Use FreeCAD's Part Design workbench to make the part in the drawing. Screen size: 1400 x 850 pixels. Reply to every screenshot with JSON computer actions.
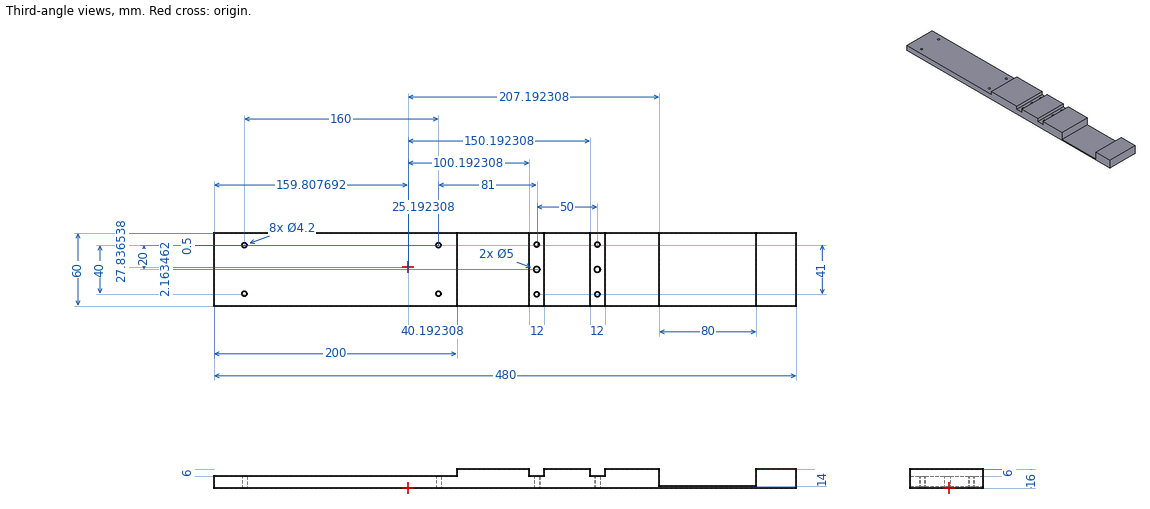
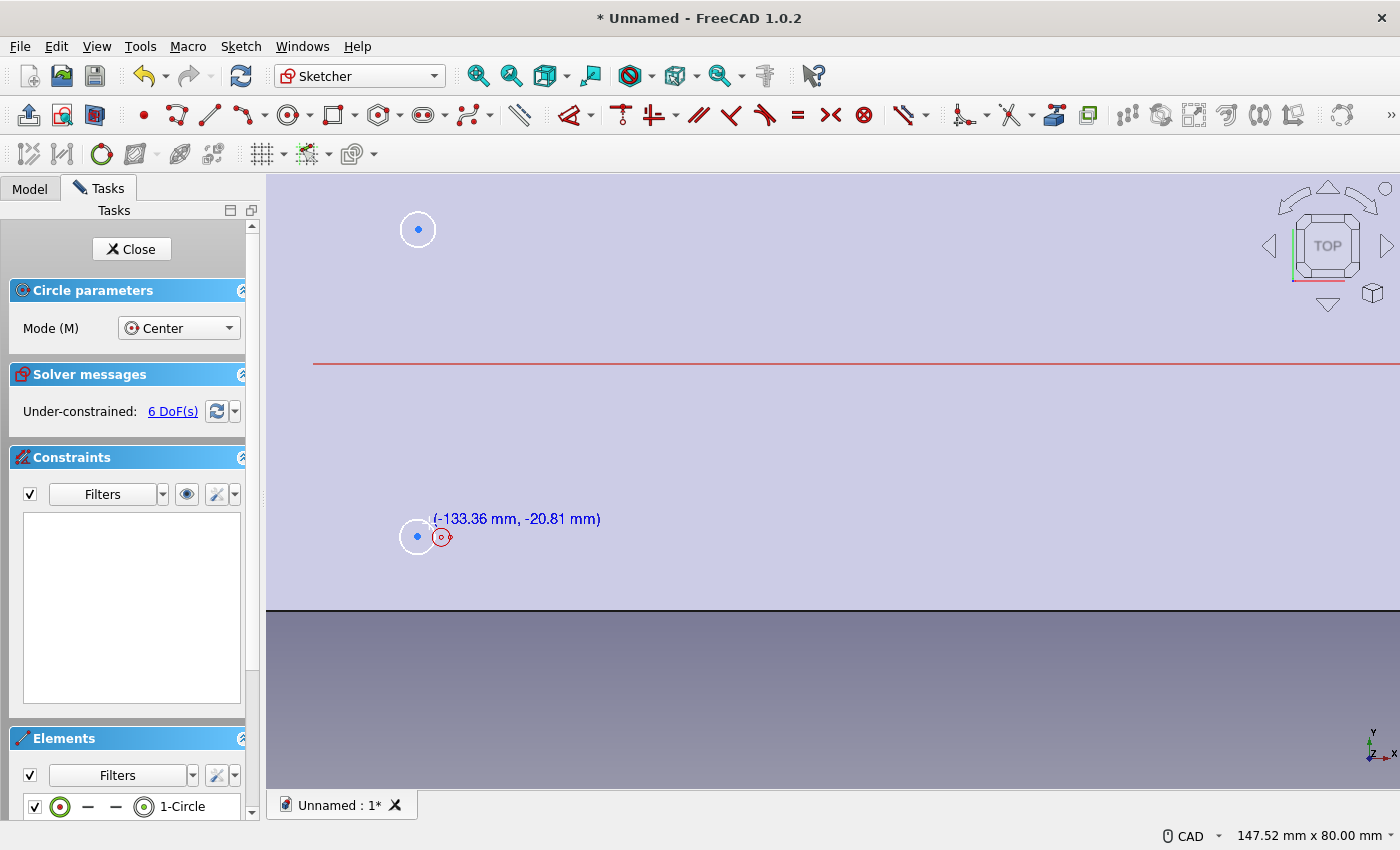
{"action": "scroll", "coordinate": [431, 525], "scroll_direction": "down", "scroll_amount": 6}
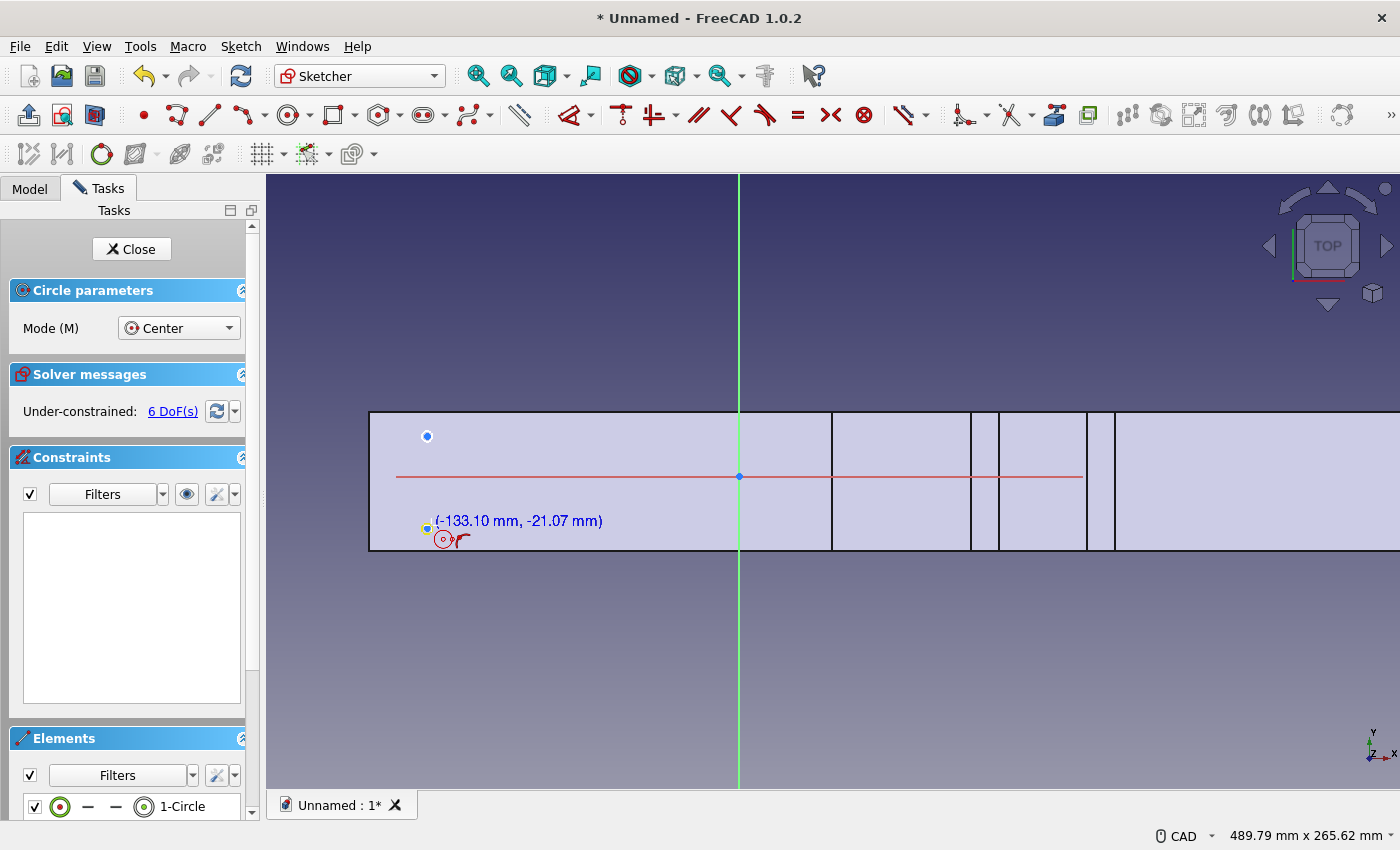
{"action": "scroll", "coordinate": [798, 436], "scroll_direction": "up", "scroll_amount": 8}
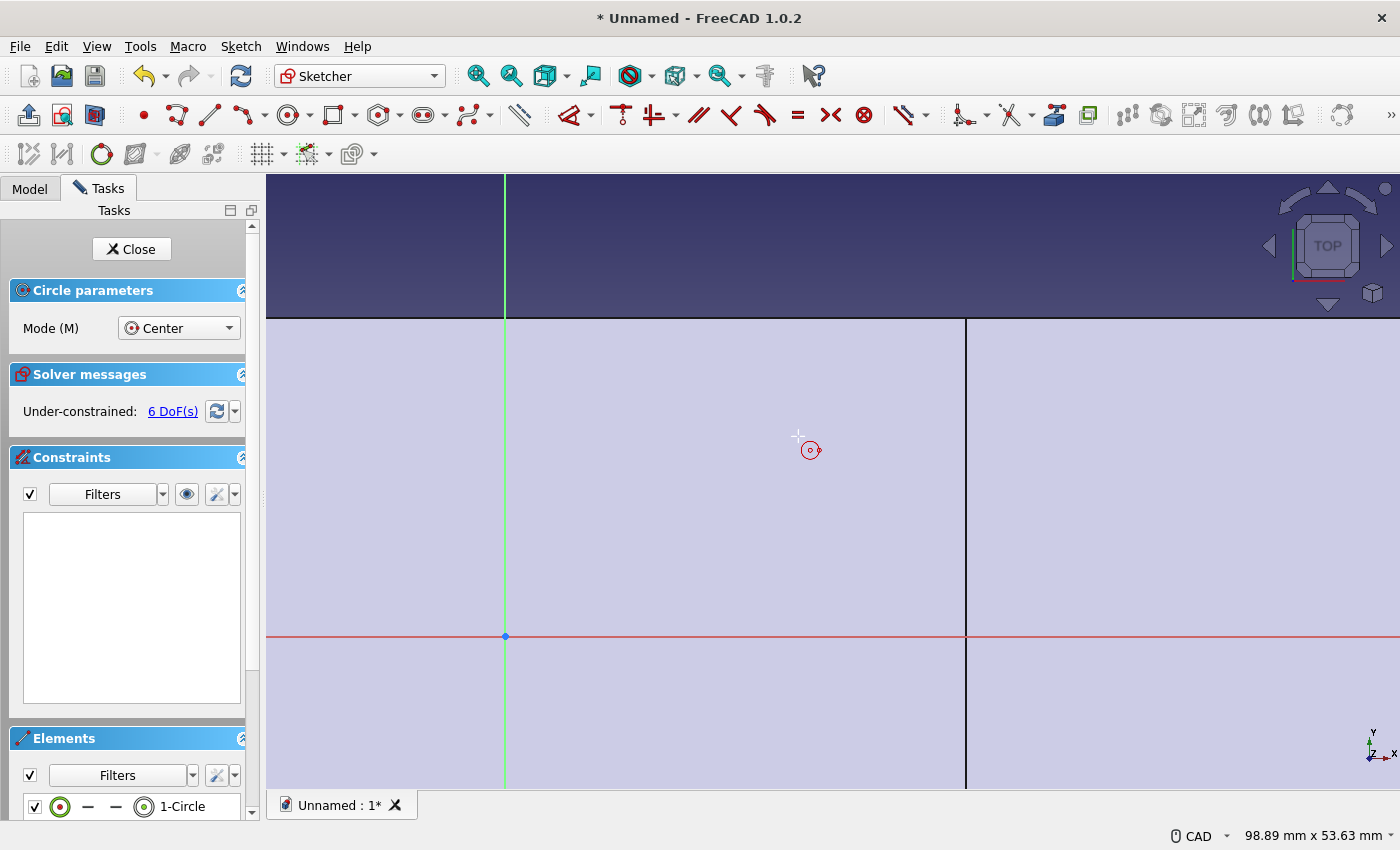
{"action": "scroll", "coordinate": [798, 436], "scroll_direction": "down", "scroll_amount": 8}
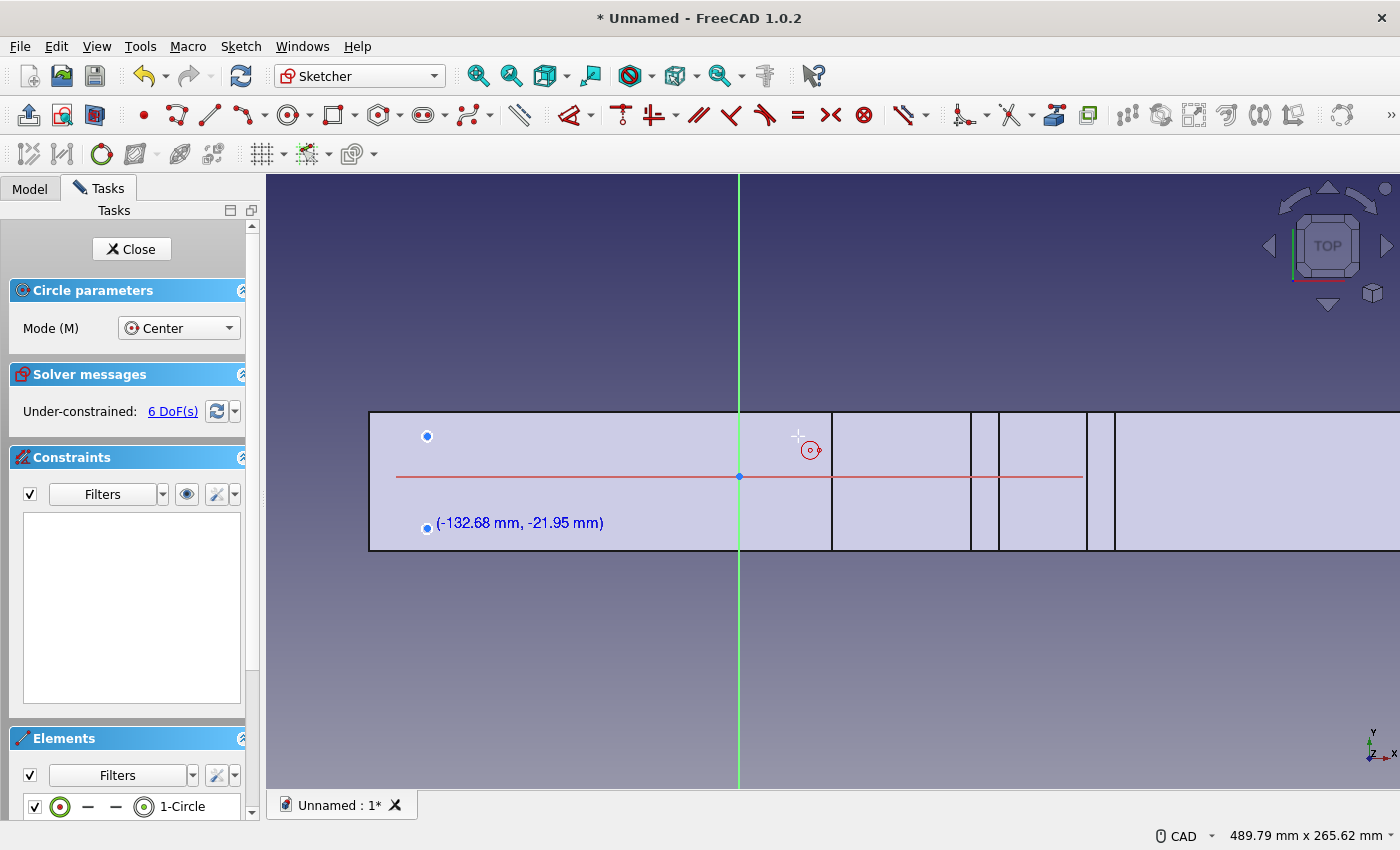
{"action": "left_click", "coordinate": [798, 436]}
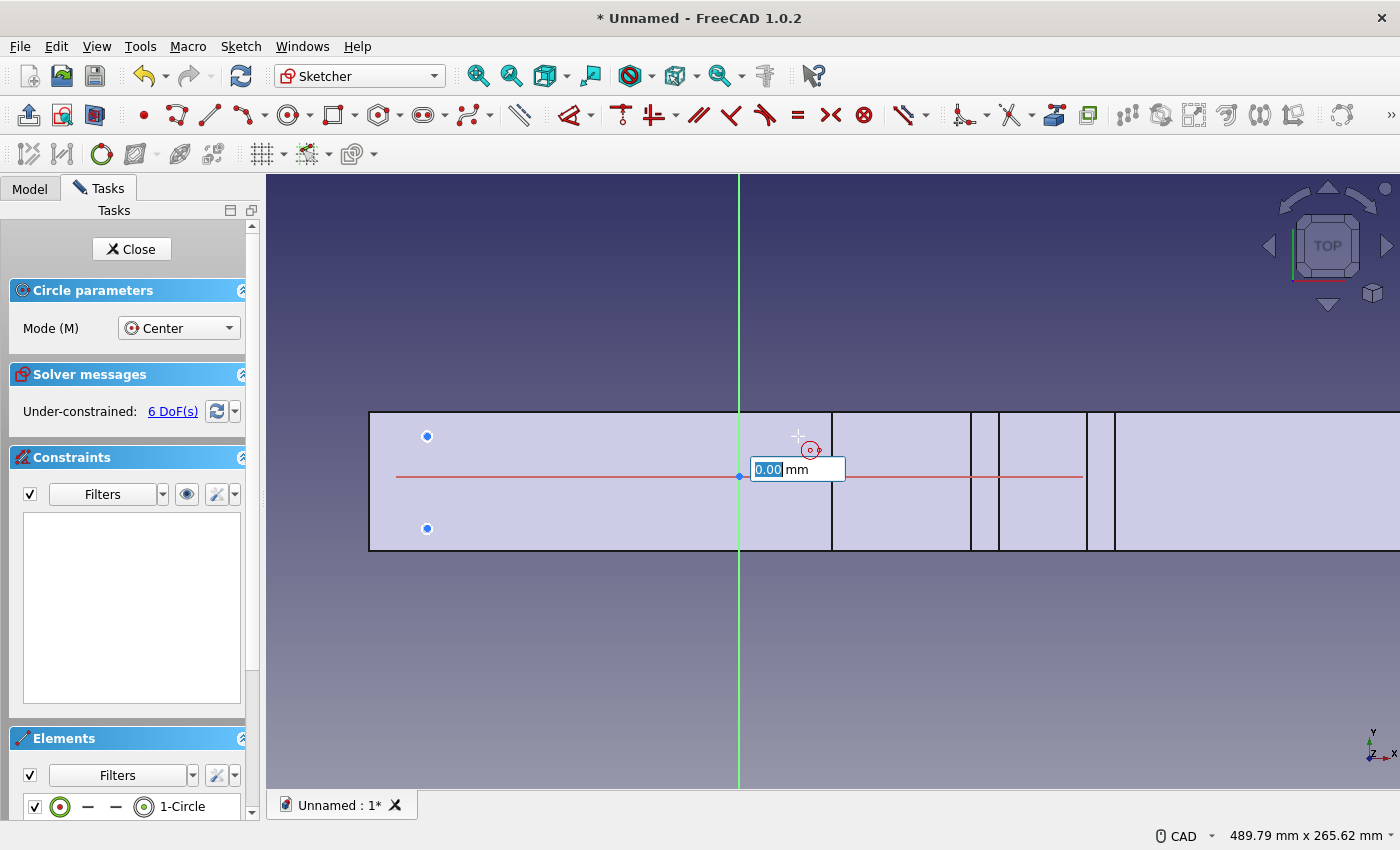
{"action": "scroll", "coordinate": [801, 432], "scroll_direction": "up", "scroll_amount": 6}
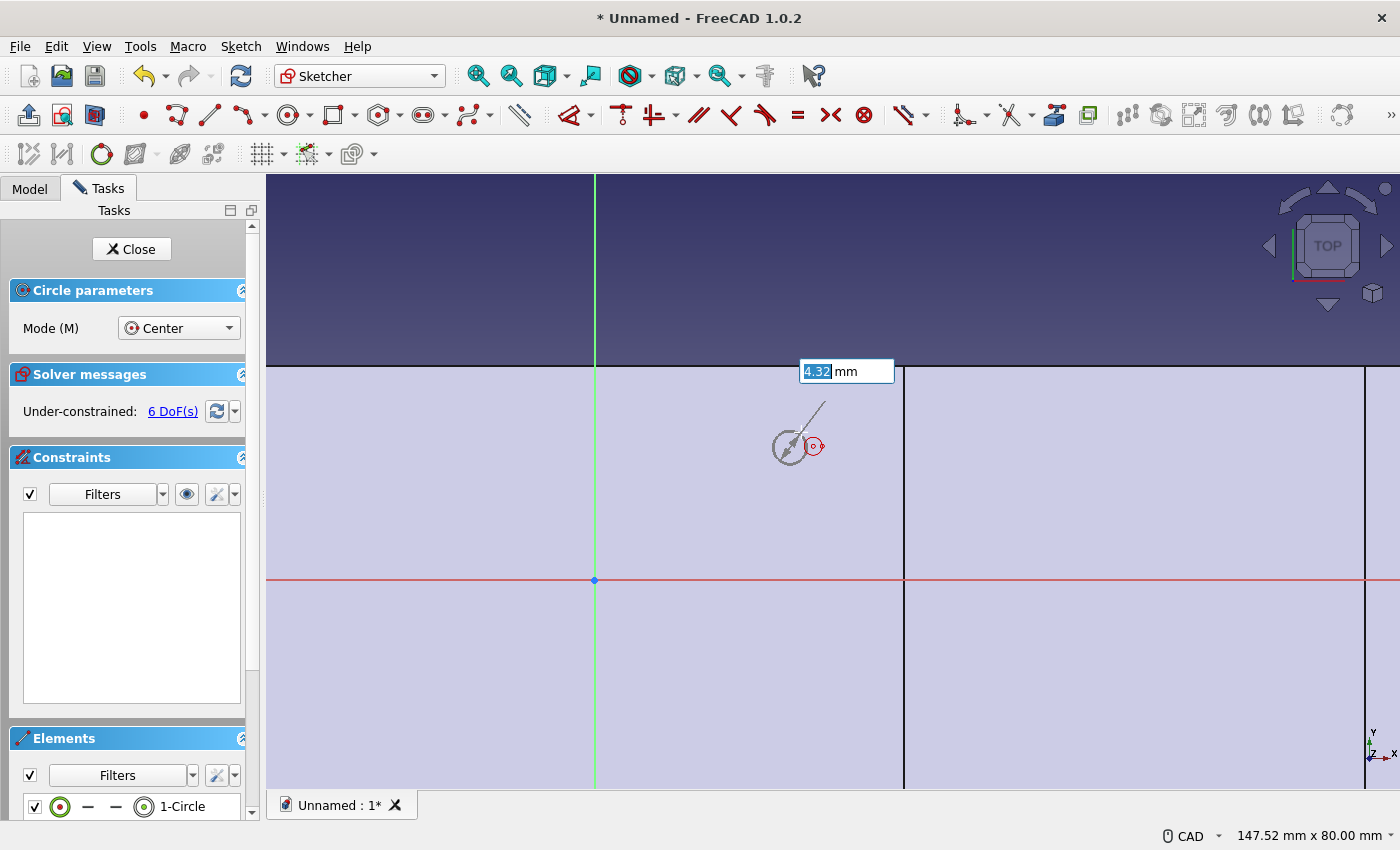
{"action": "left_click", "coordinate": [800, 432]}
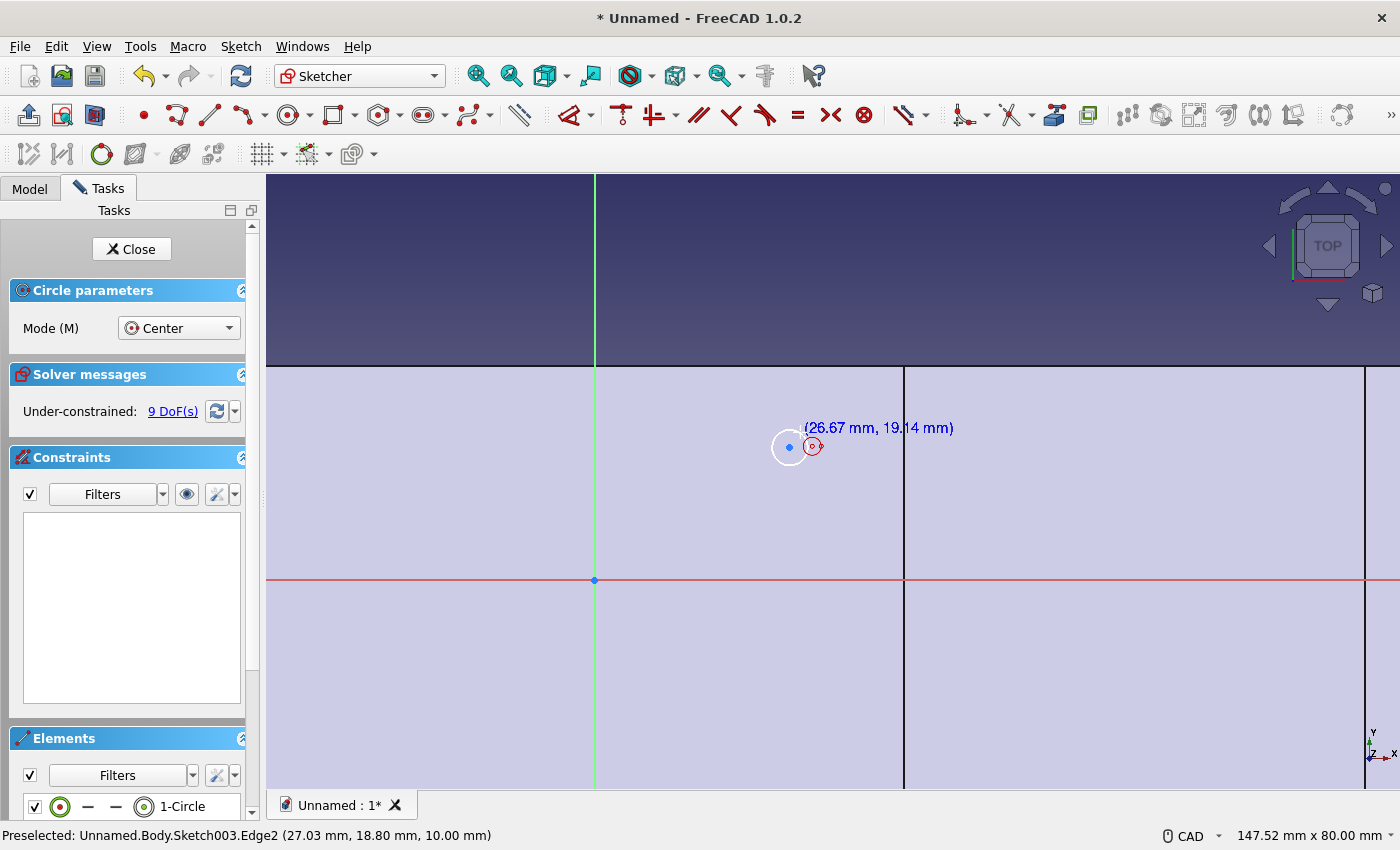
{"action": "scroll", "coordinate": [789, 751], "scroll_direction": "up", "scroll_amount": 2}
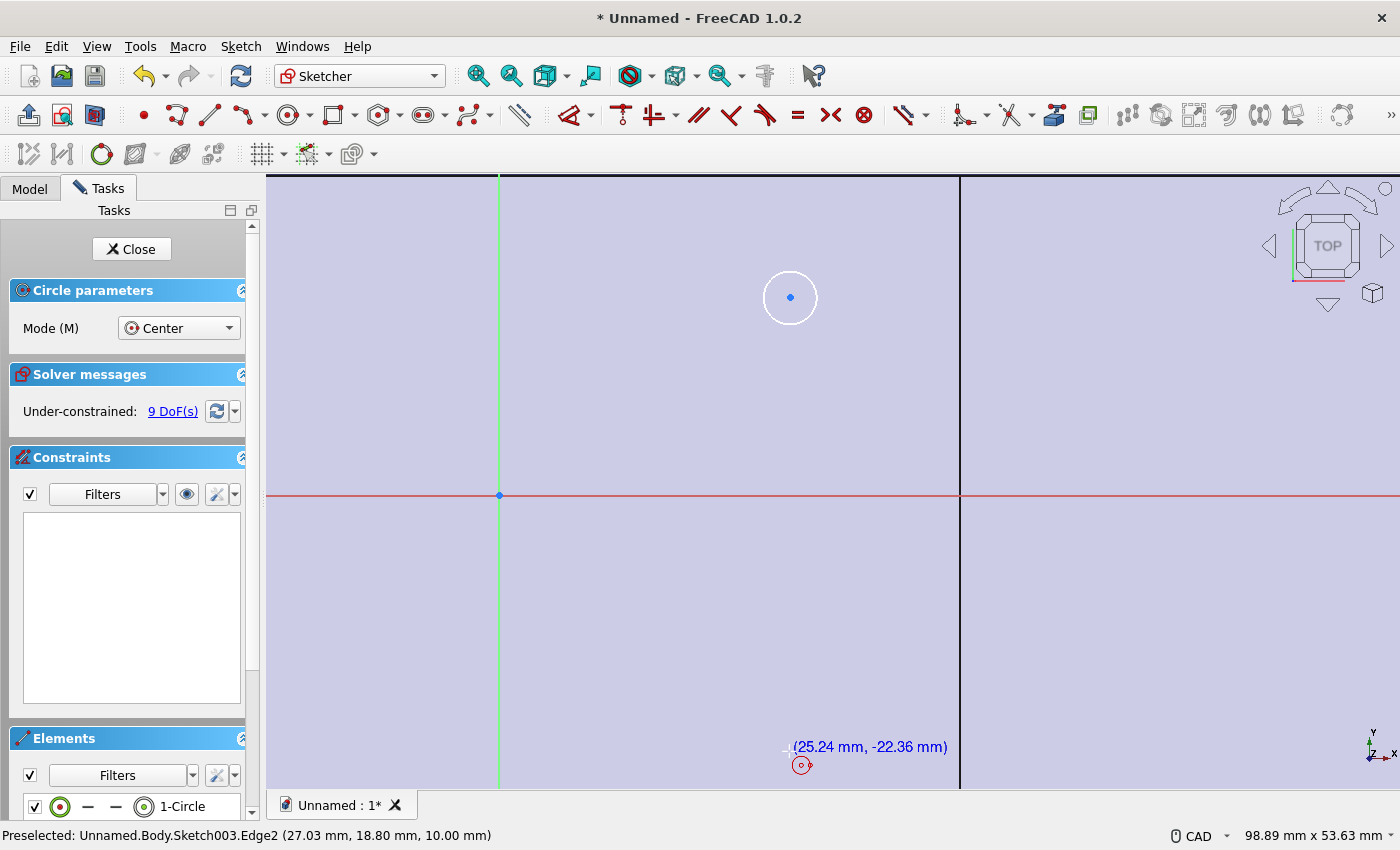
{"action": "scroll", "coordinate": [800, 472], "scroll_direction": "down", "scroll_amount": 8}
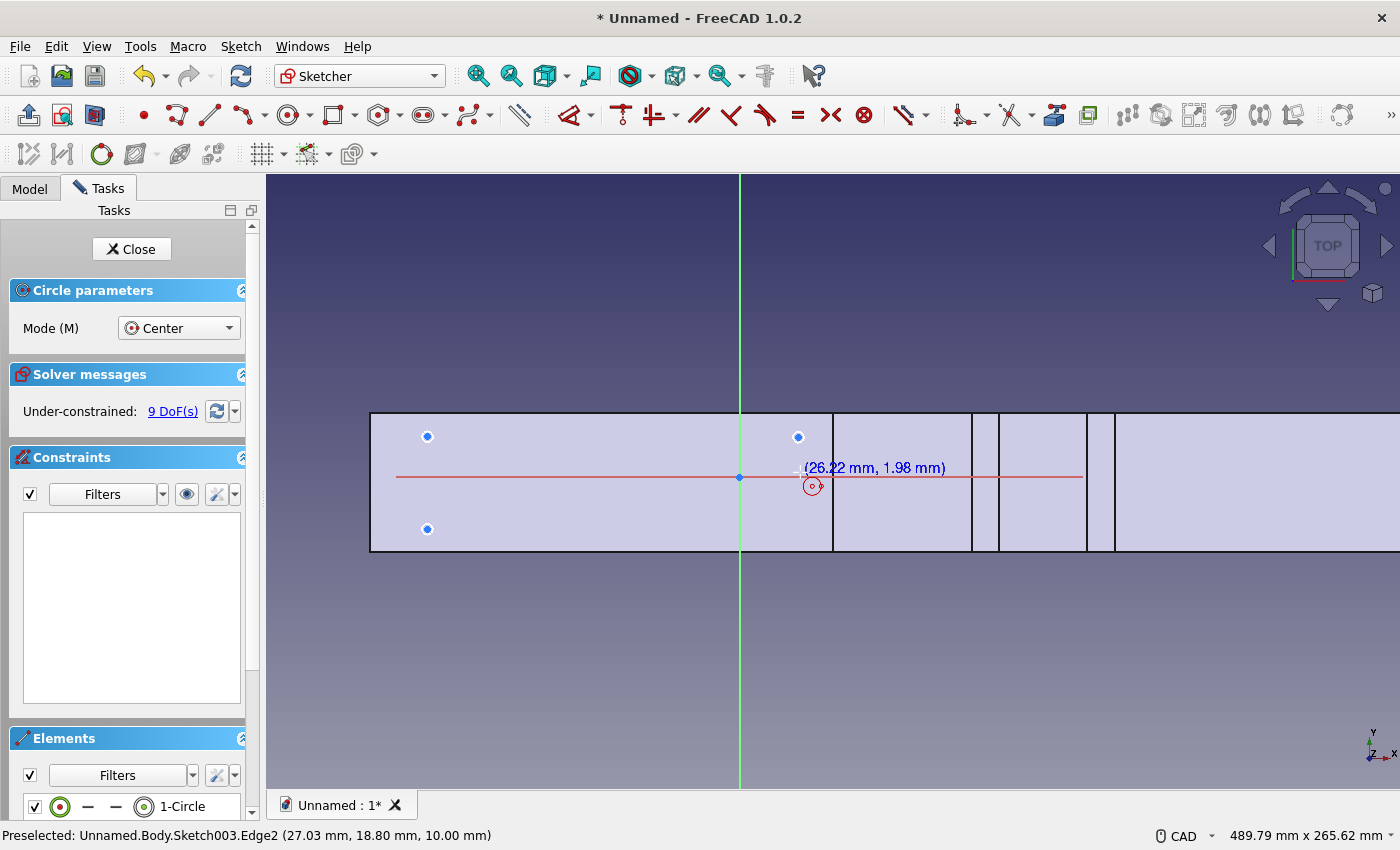
{"action": "left_click", "coordinate": [798, 528]}